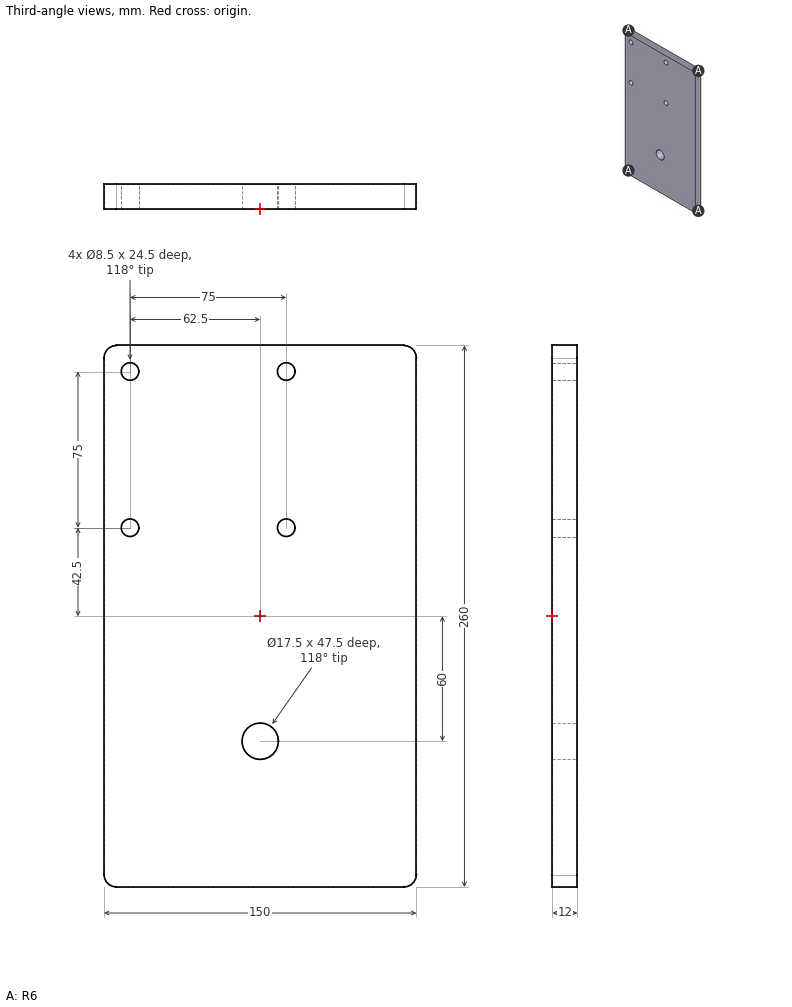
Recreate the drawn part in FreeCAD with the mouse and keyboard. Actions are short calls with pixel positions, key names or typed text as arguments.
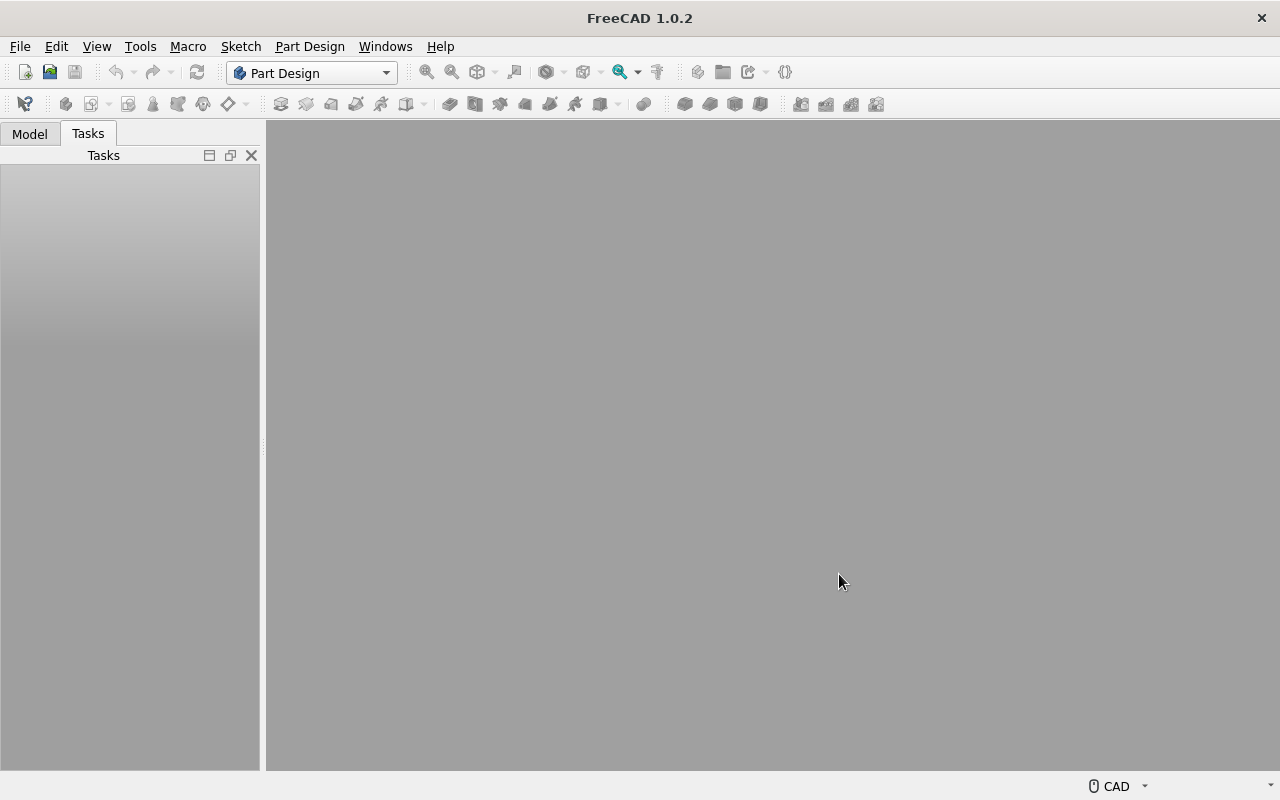
key(ctrl+n)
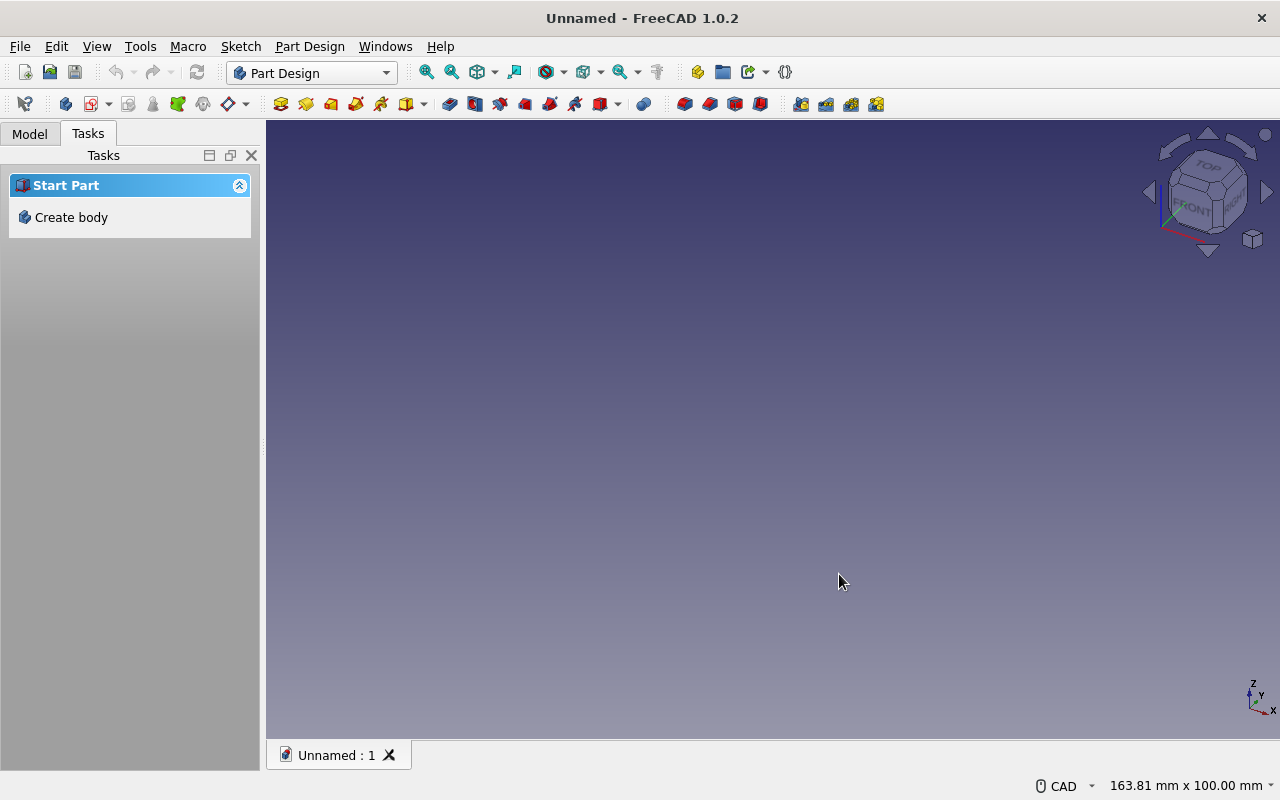
click(90, 104)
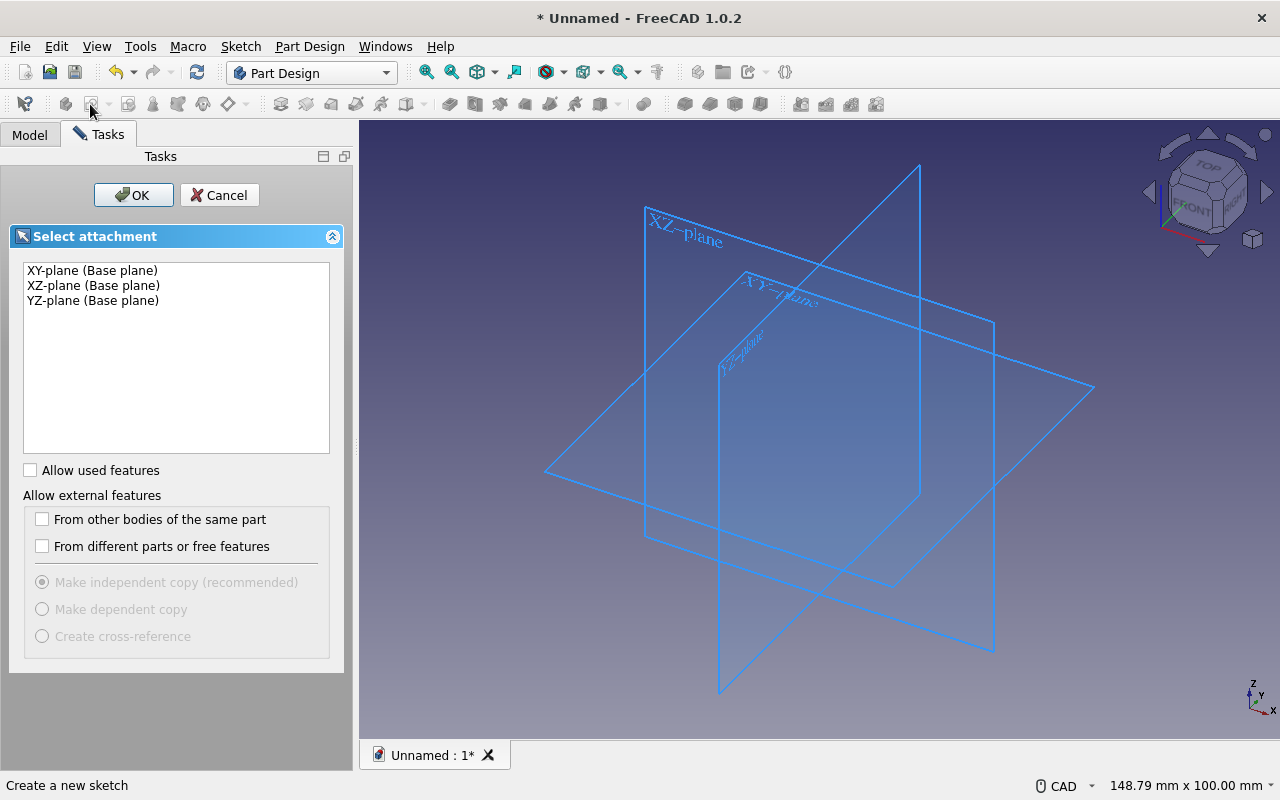
click(84, 286)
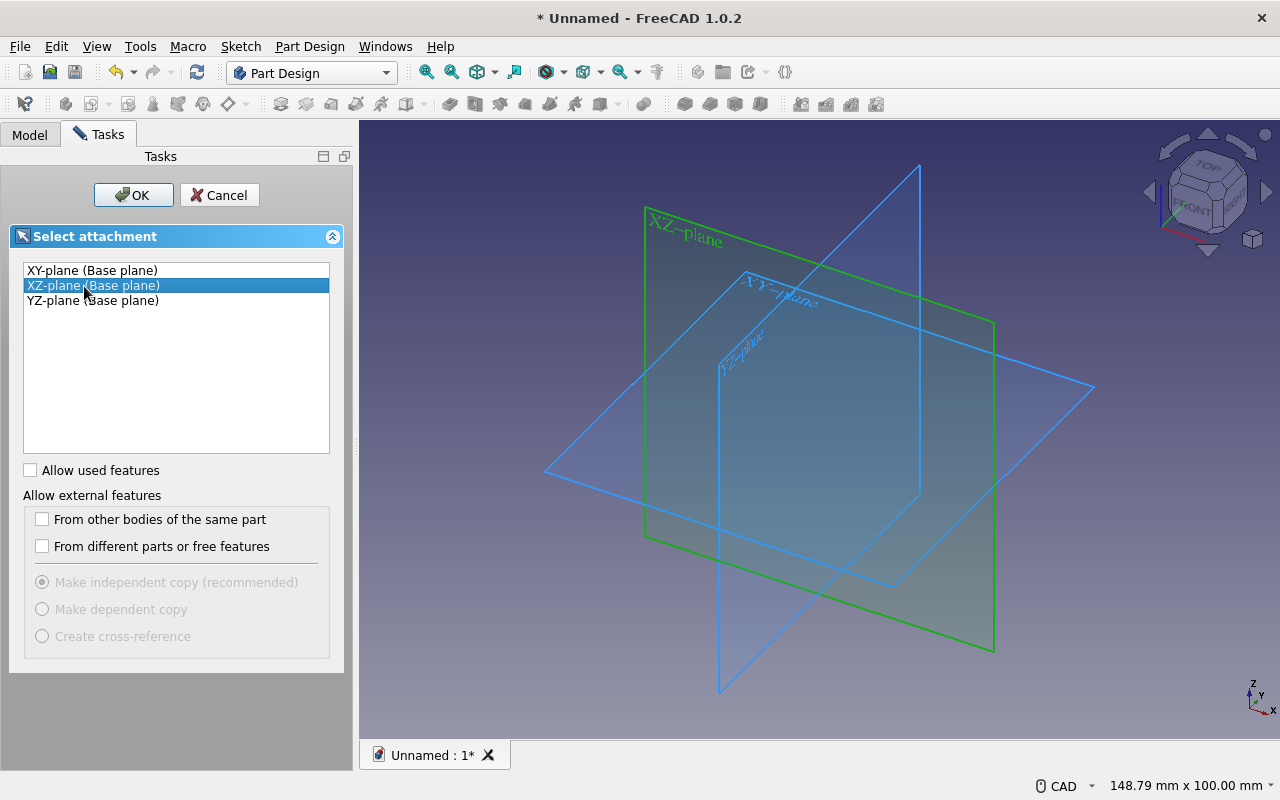
click(134, 195)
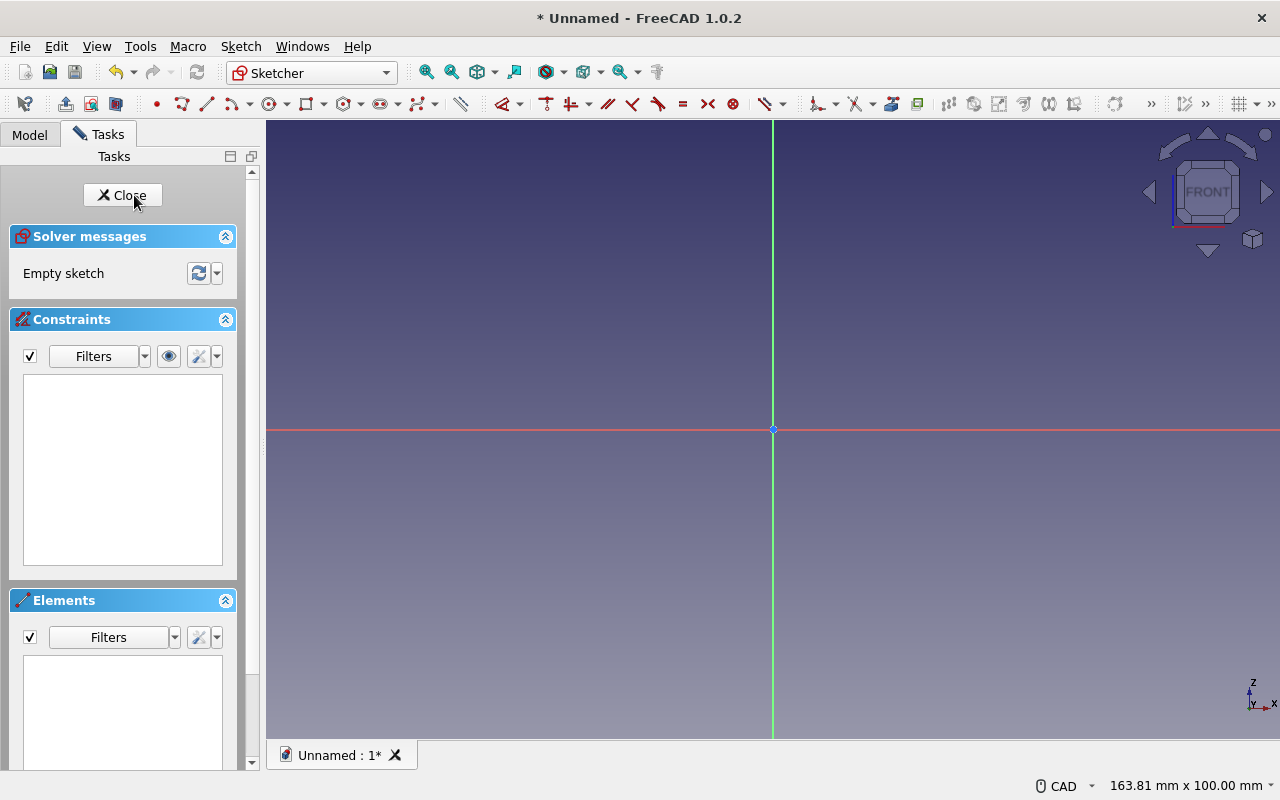
scroll(682, 430, down, 7)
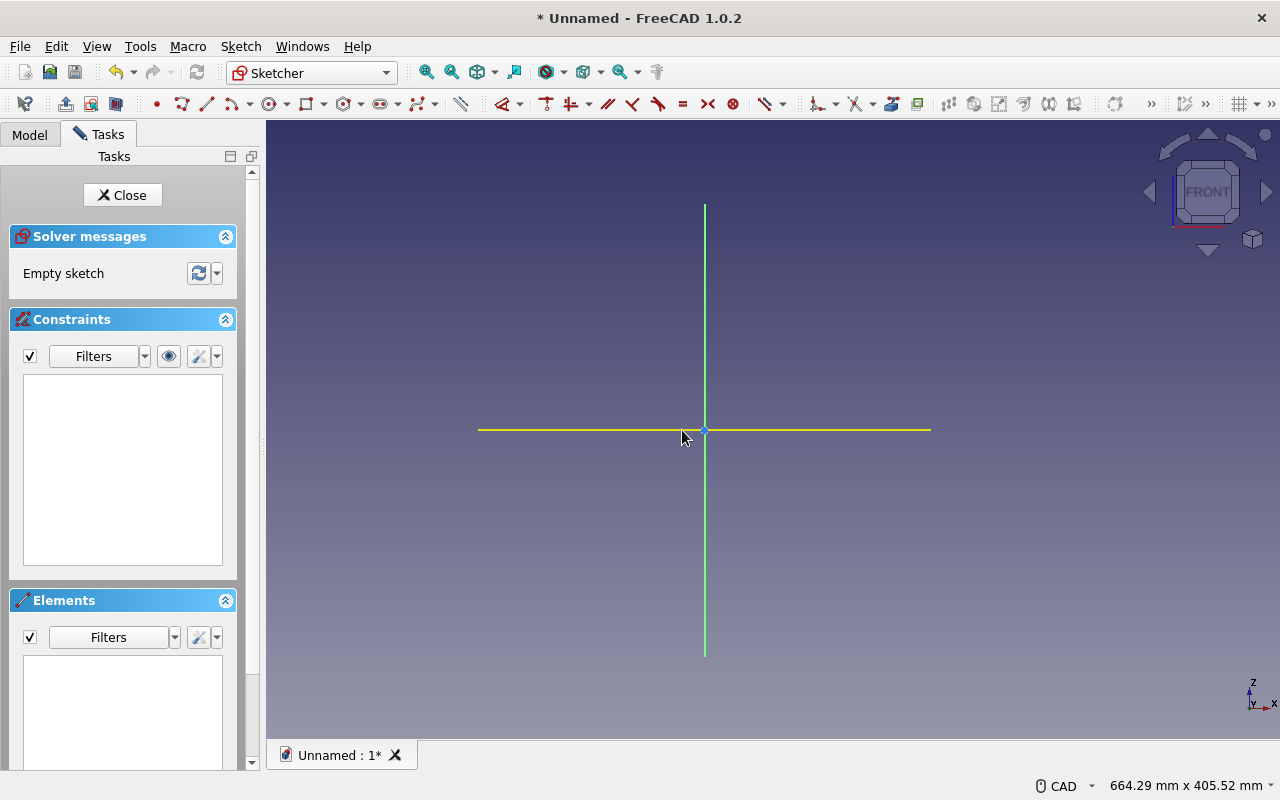
key(g)
key(v)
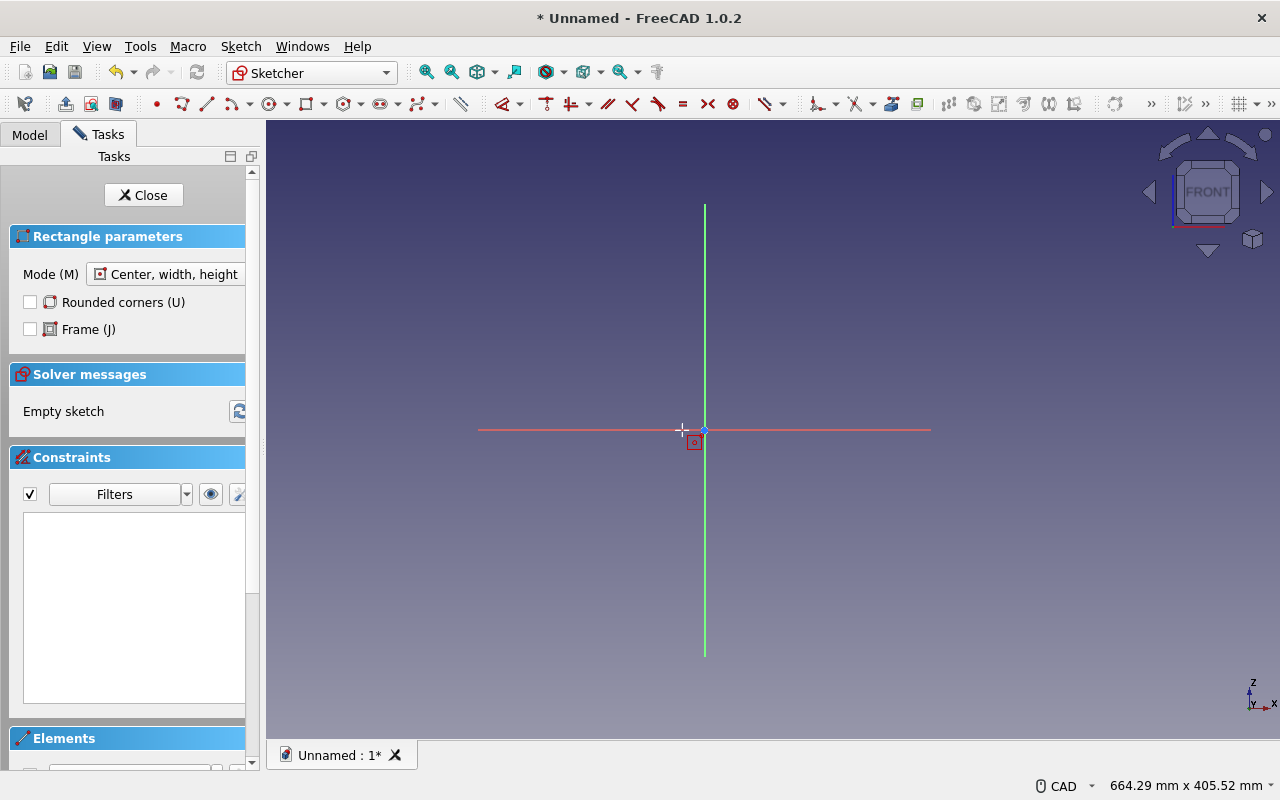
click(705, 430)
move(819, 232)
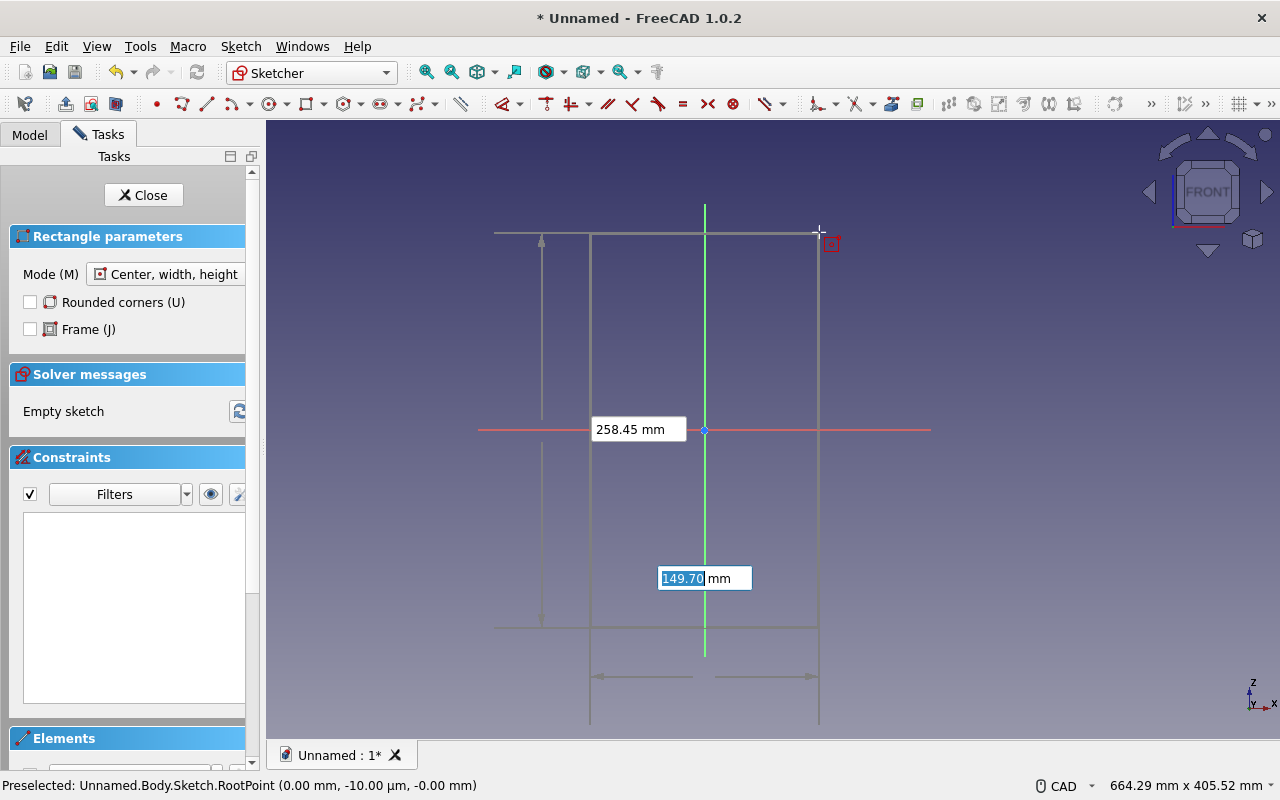
text(150)
key(Tab)
text(260)
key(Return)
key(Escape)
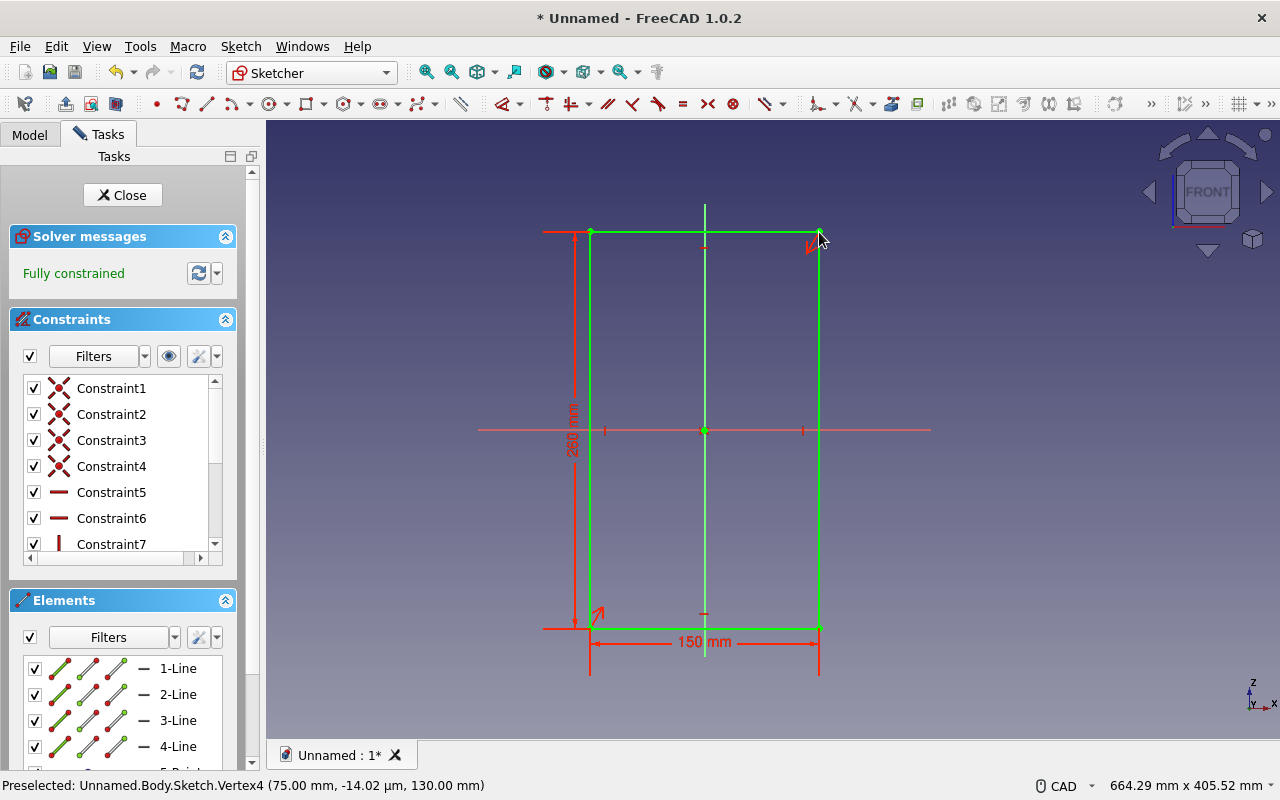
click(123, 195)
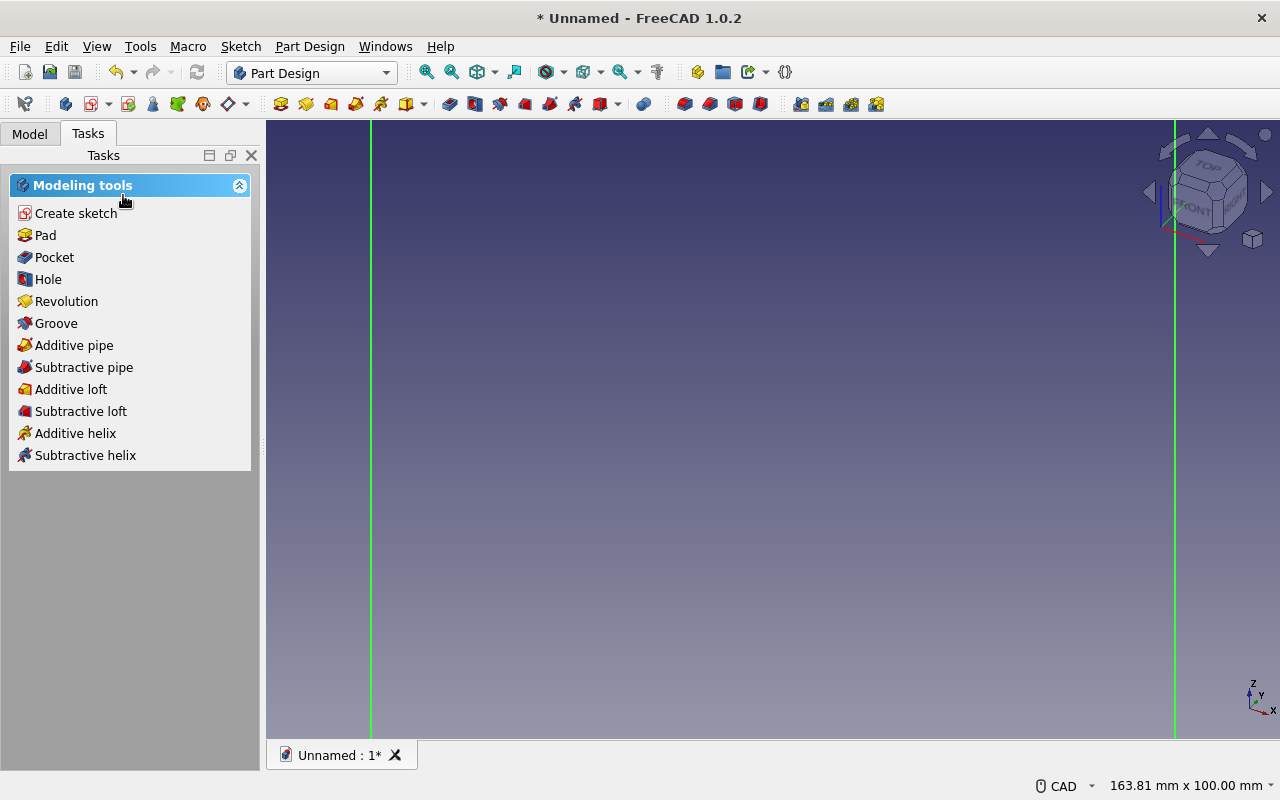
click(281, 104)